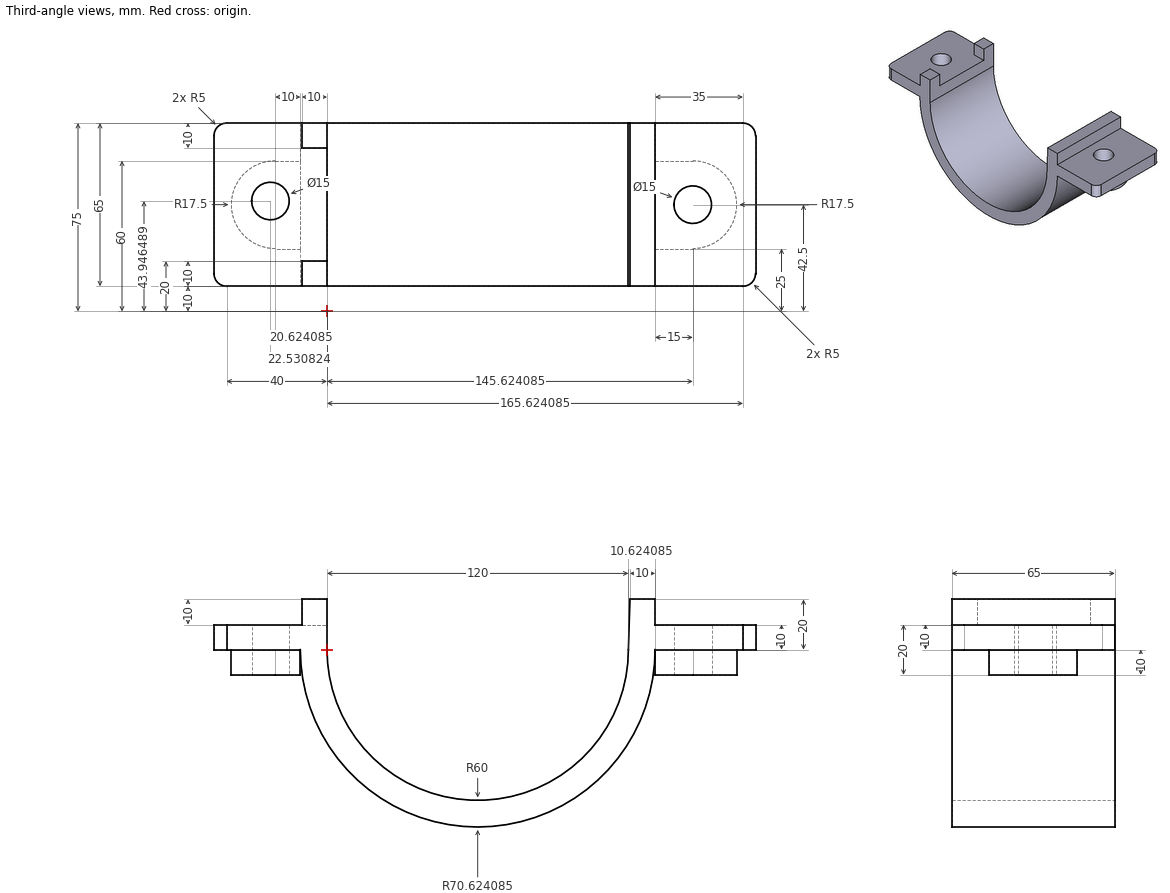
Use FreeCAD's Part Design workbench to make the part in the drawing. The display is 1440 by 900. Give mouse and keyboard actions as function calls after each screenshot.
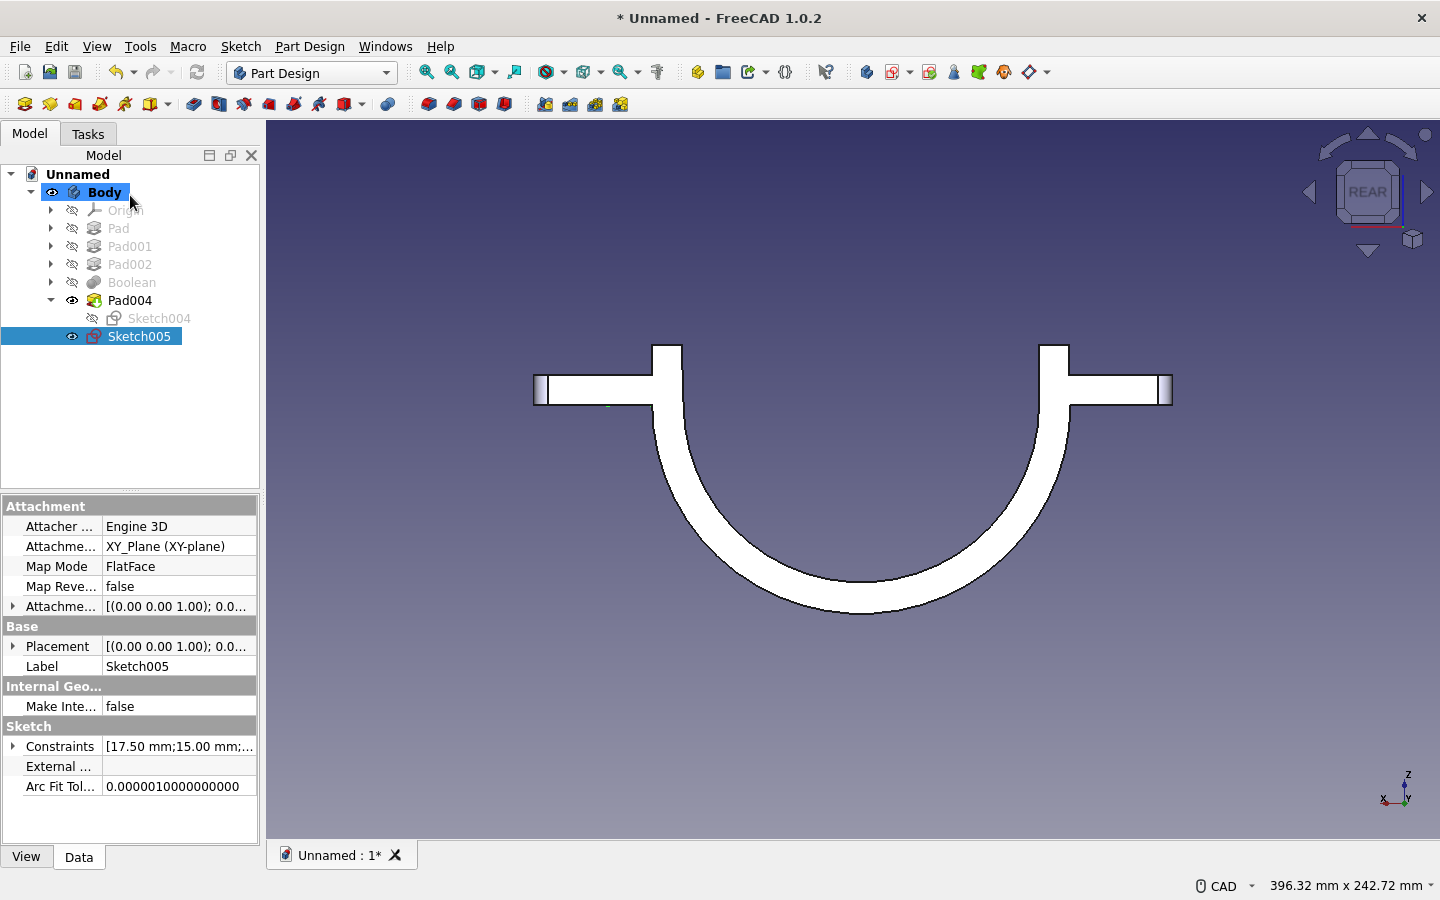
click(25, 104)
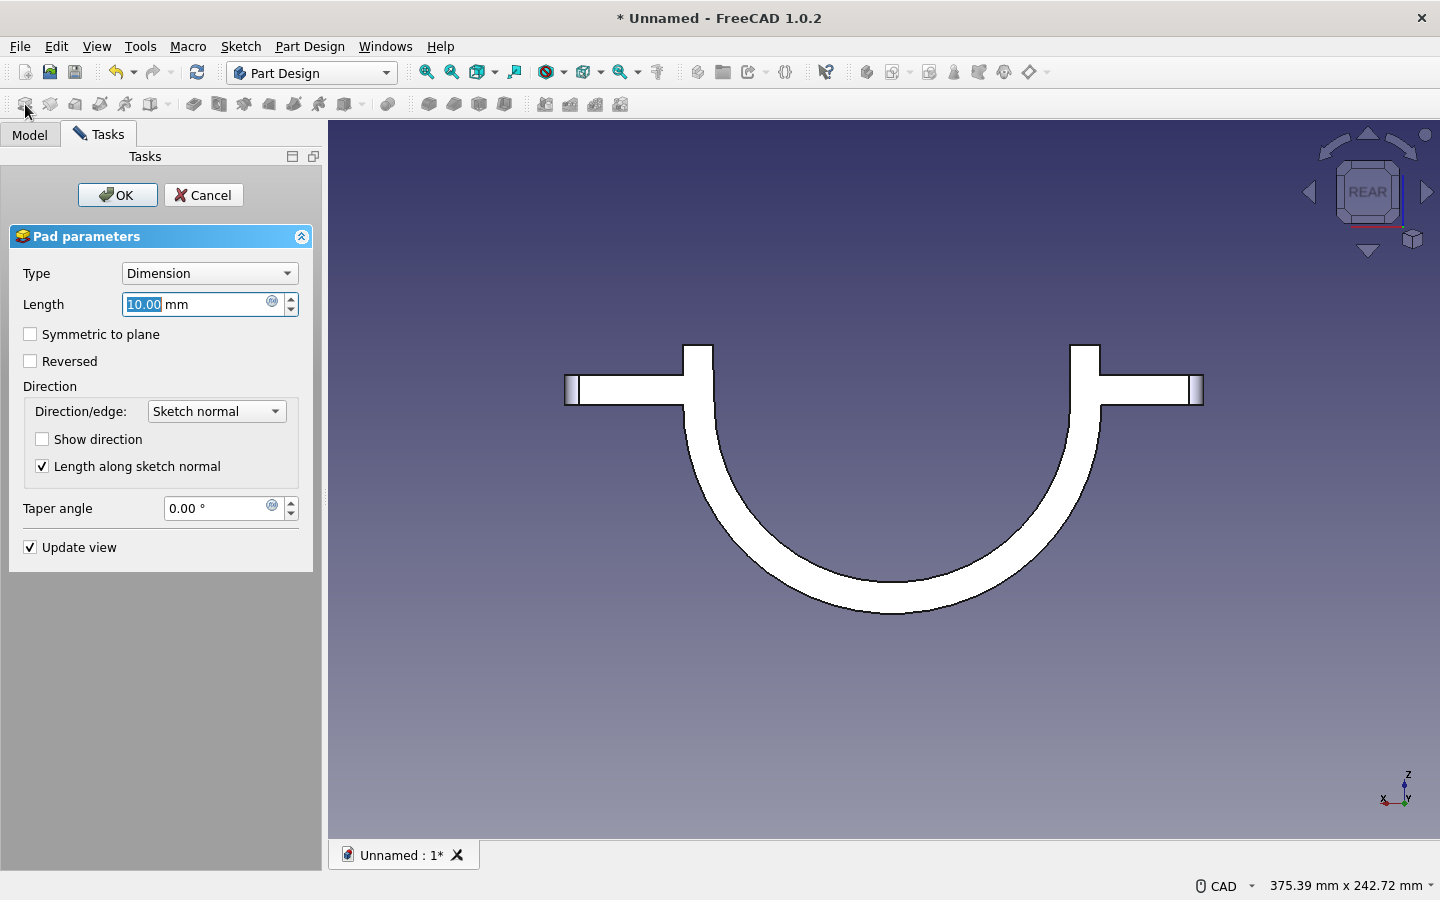
text(10)
key(Tab)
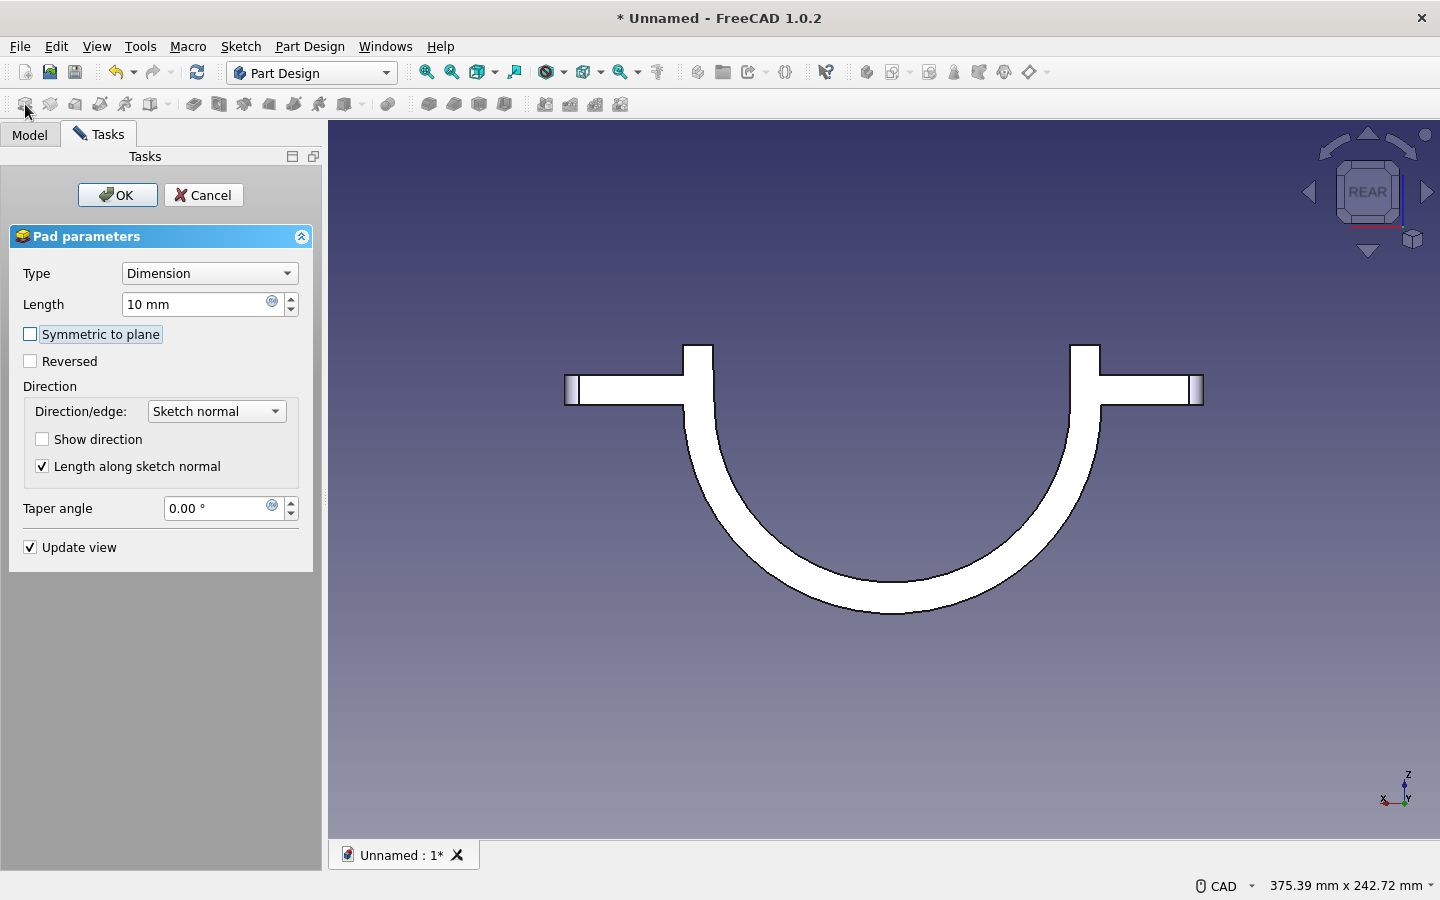
click(31, 361)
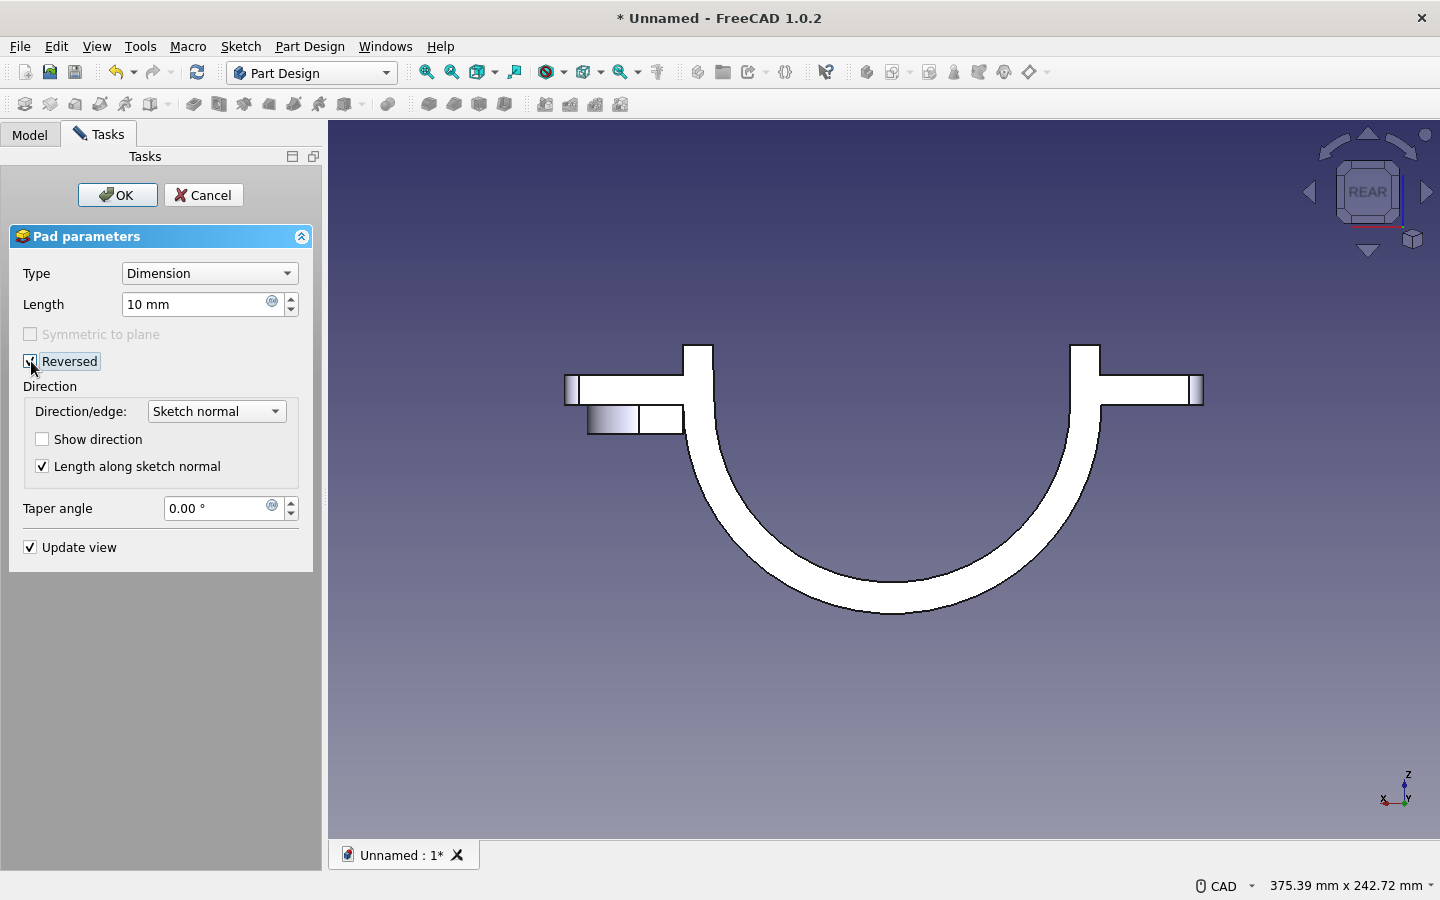
click(118, 195)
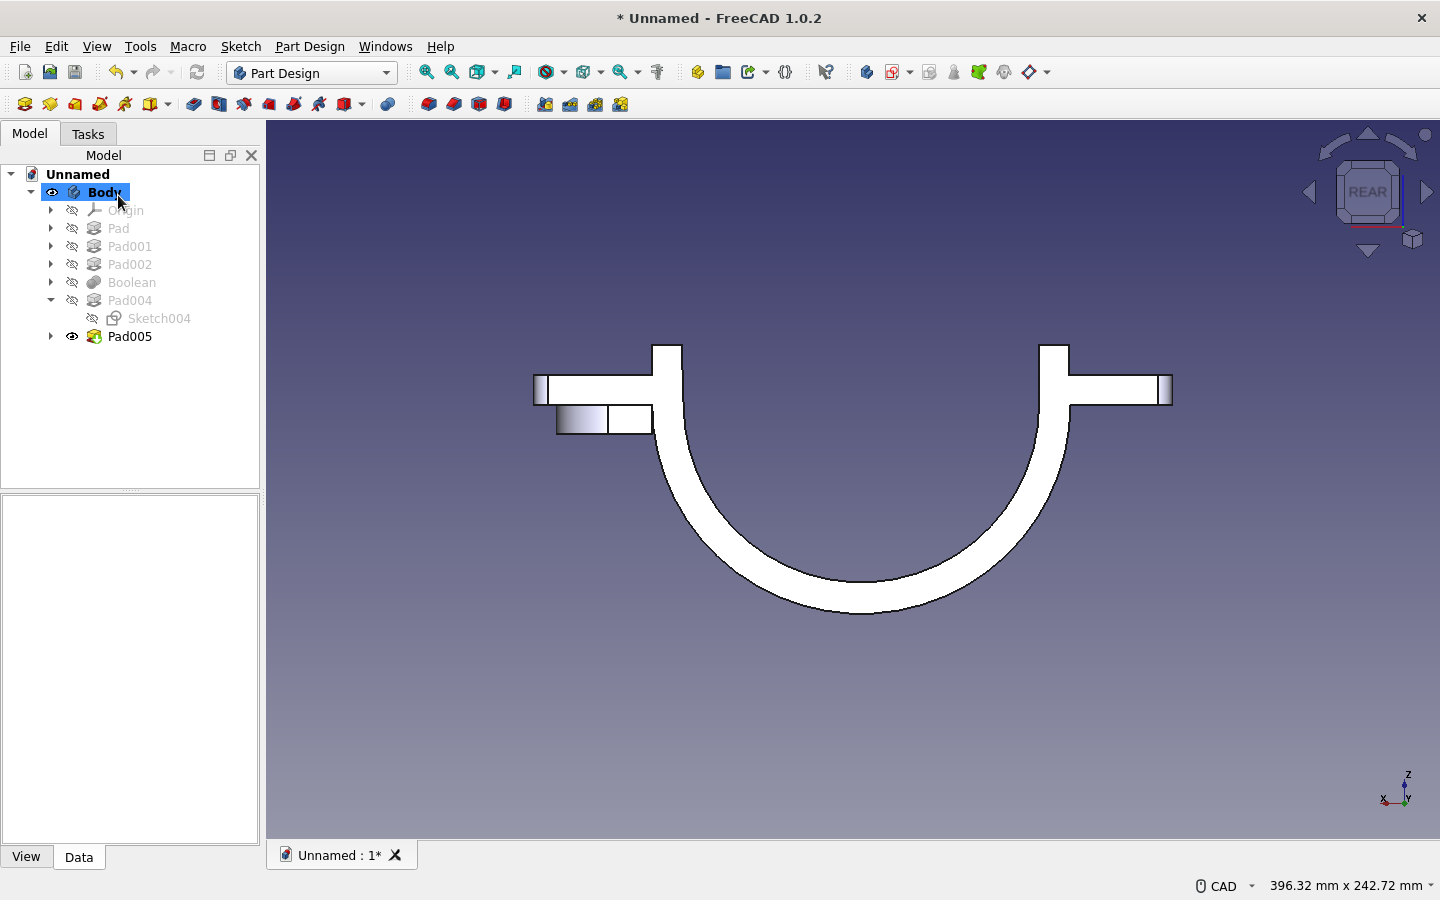
click(892, 72)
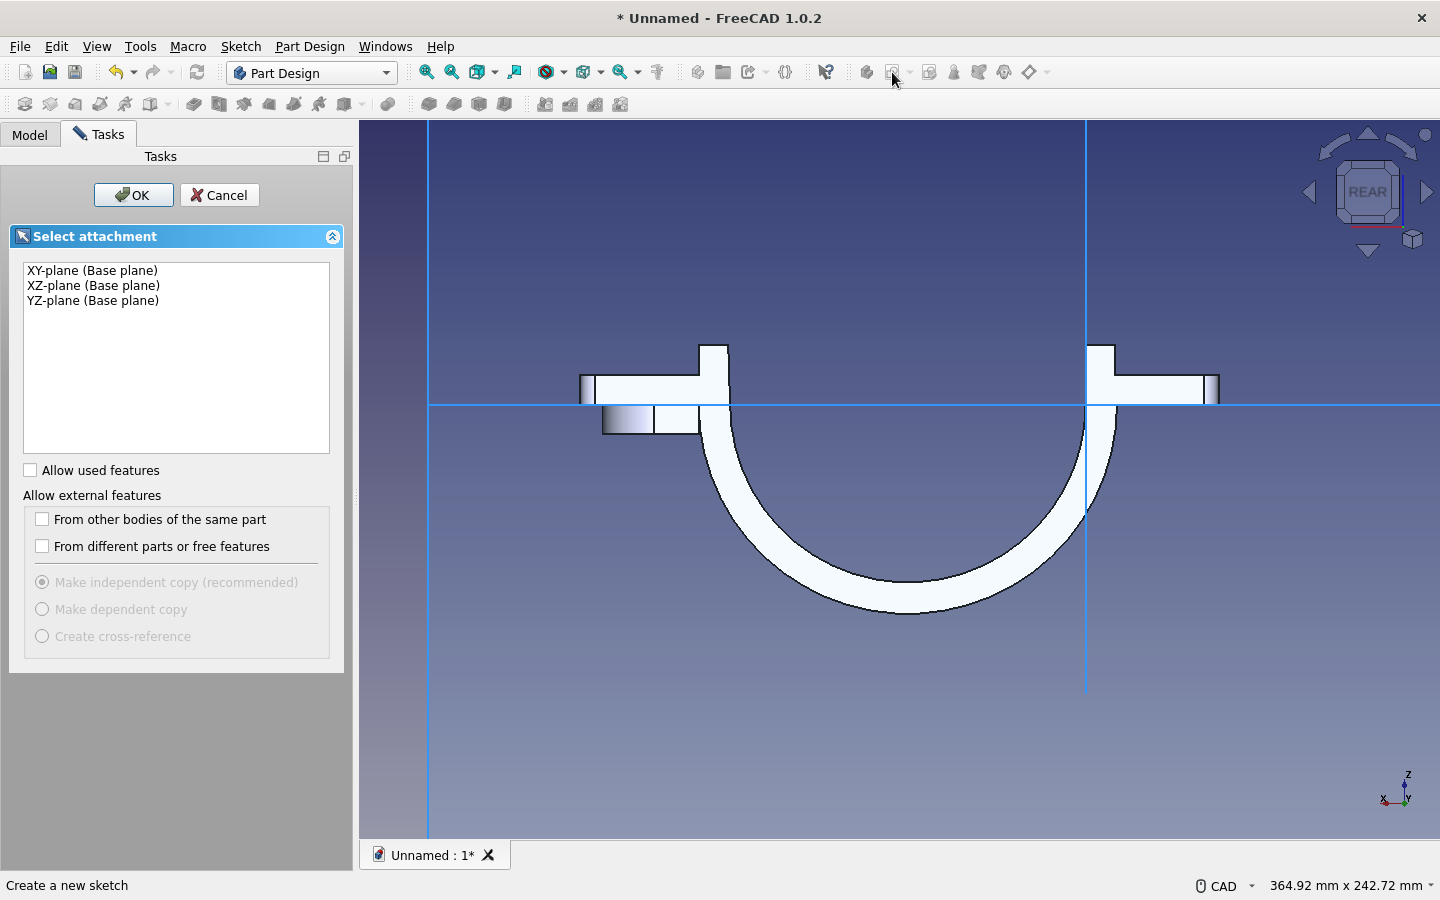
click(84, 270)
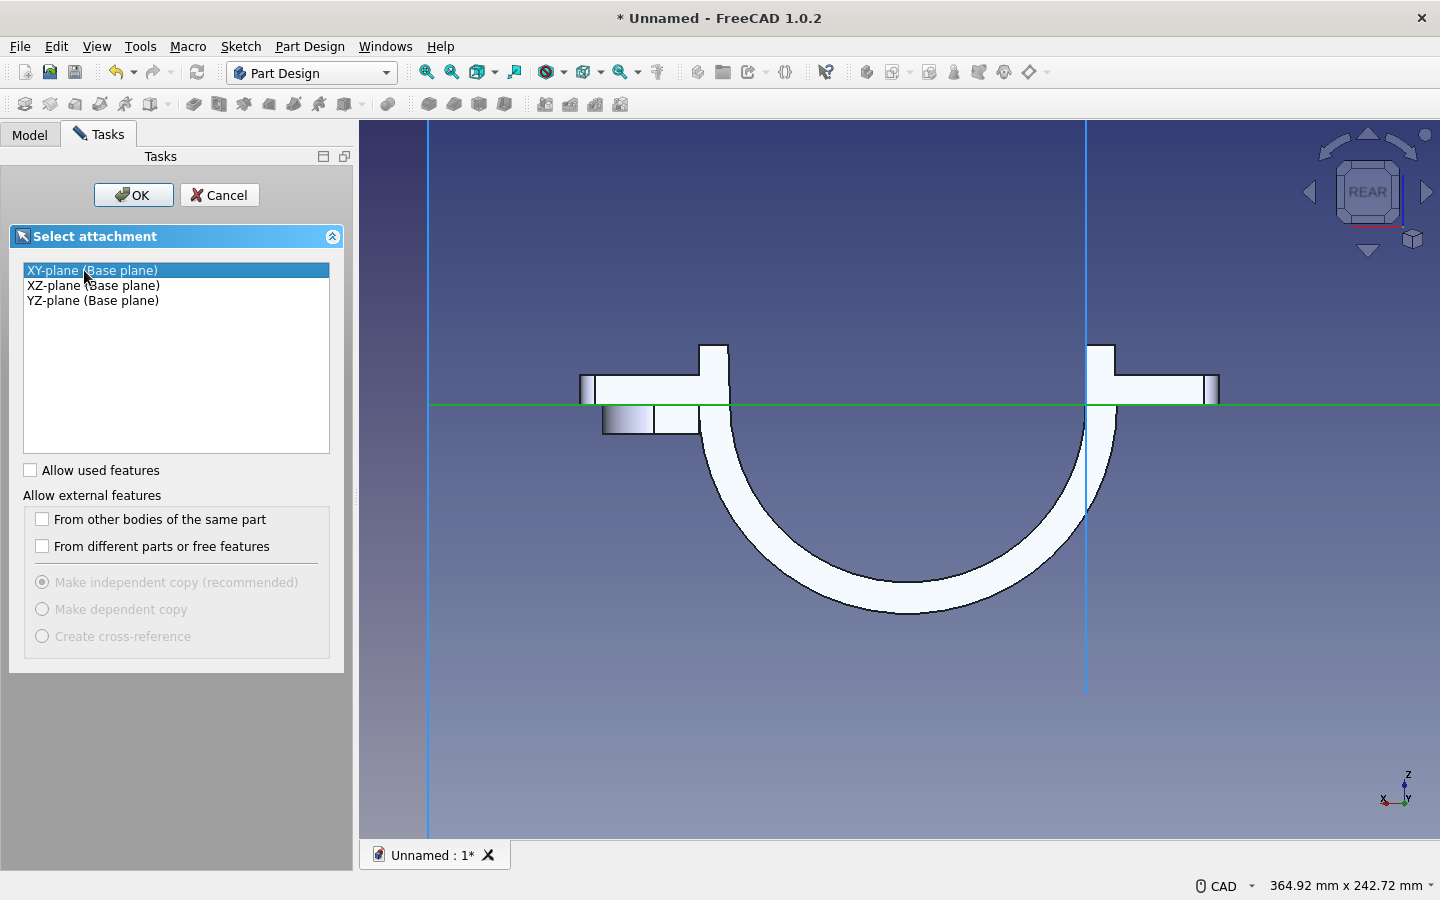
click(134, 195)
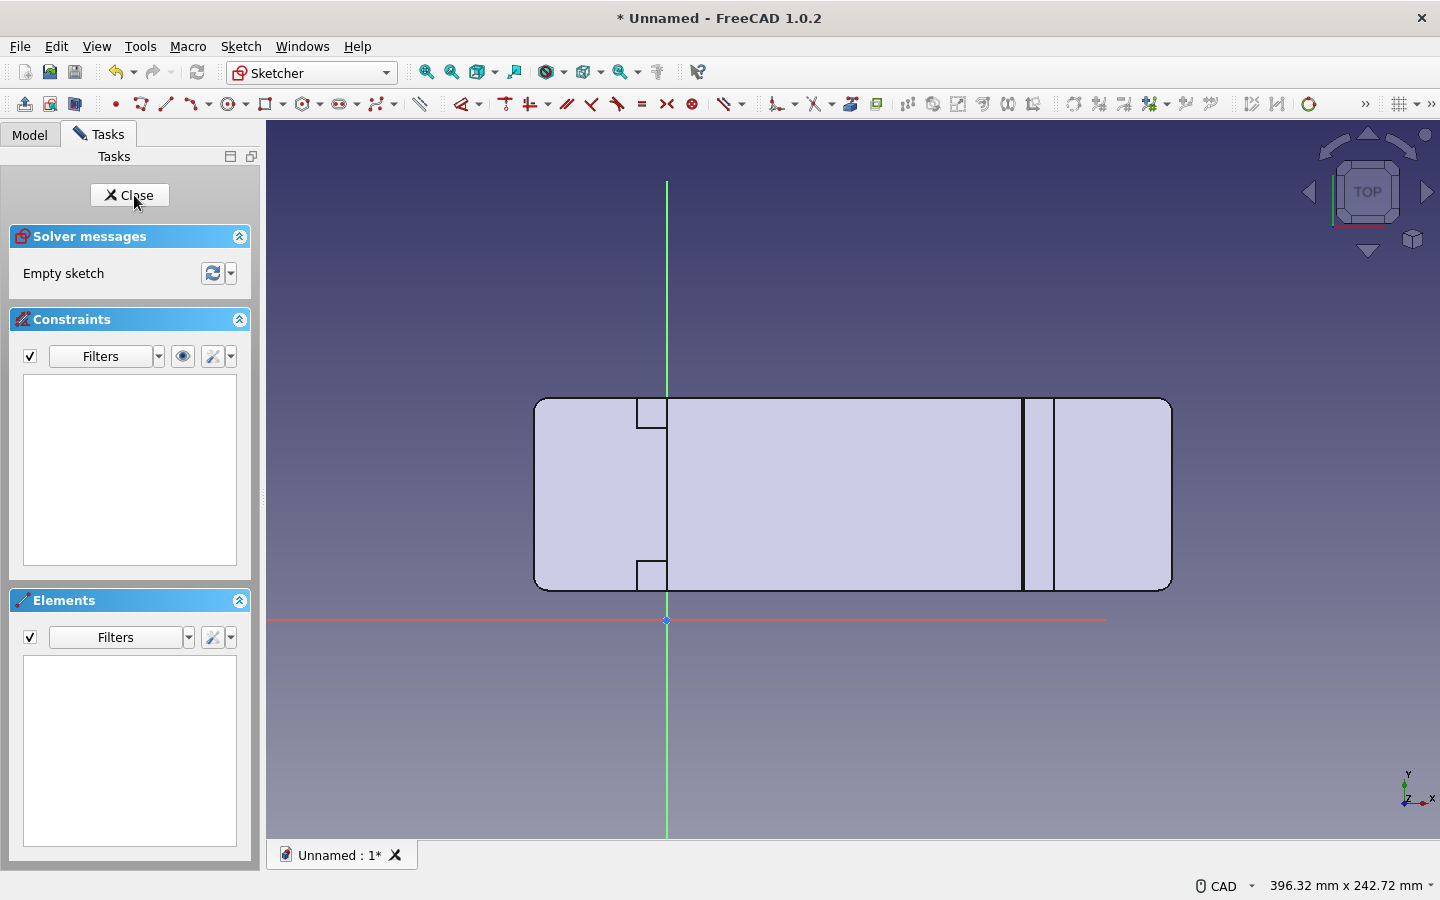
key(q)
key(s)